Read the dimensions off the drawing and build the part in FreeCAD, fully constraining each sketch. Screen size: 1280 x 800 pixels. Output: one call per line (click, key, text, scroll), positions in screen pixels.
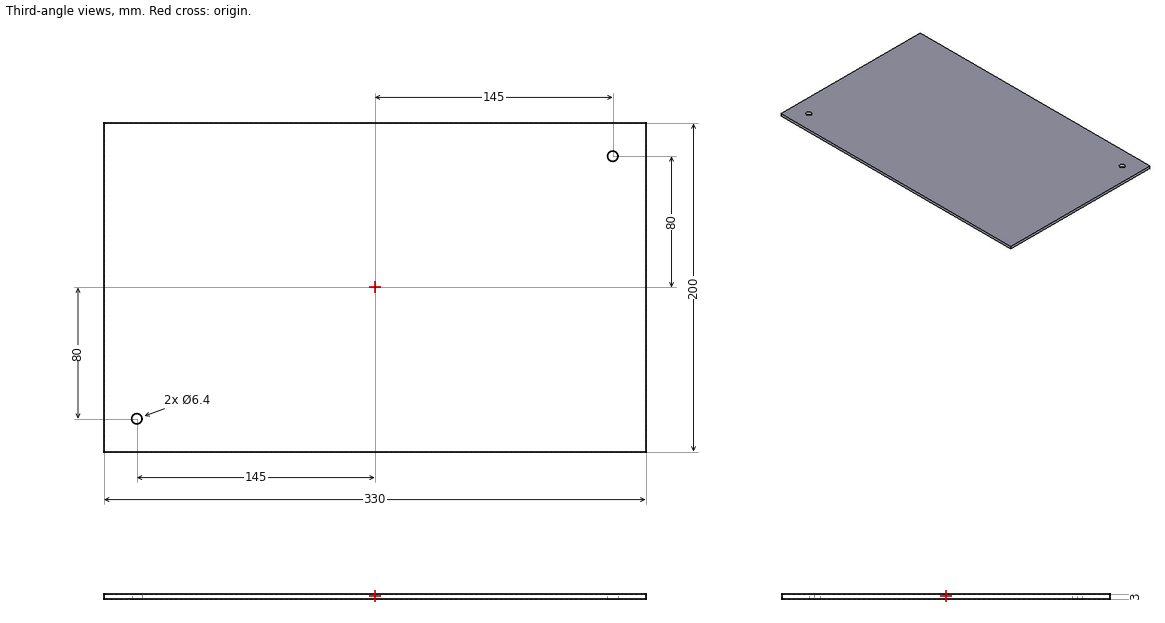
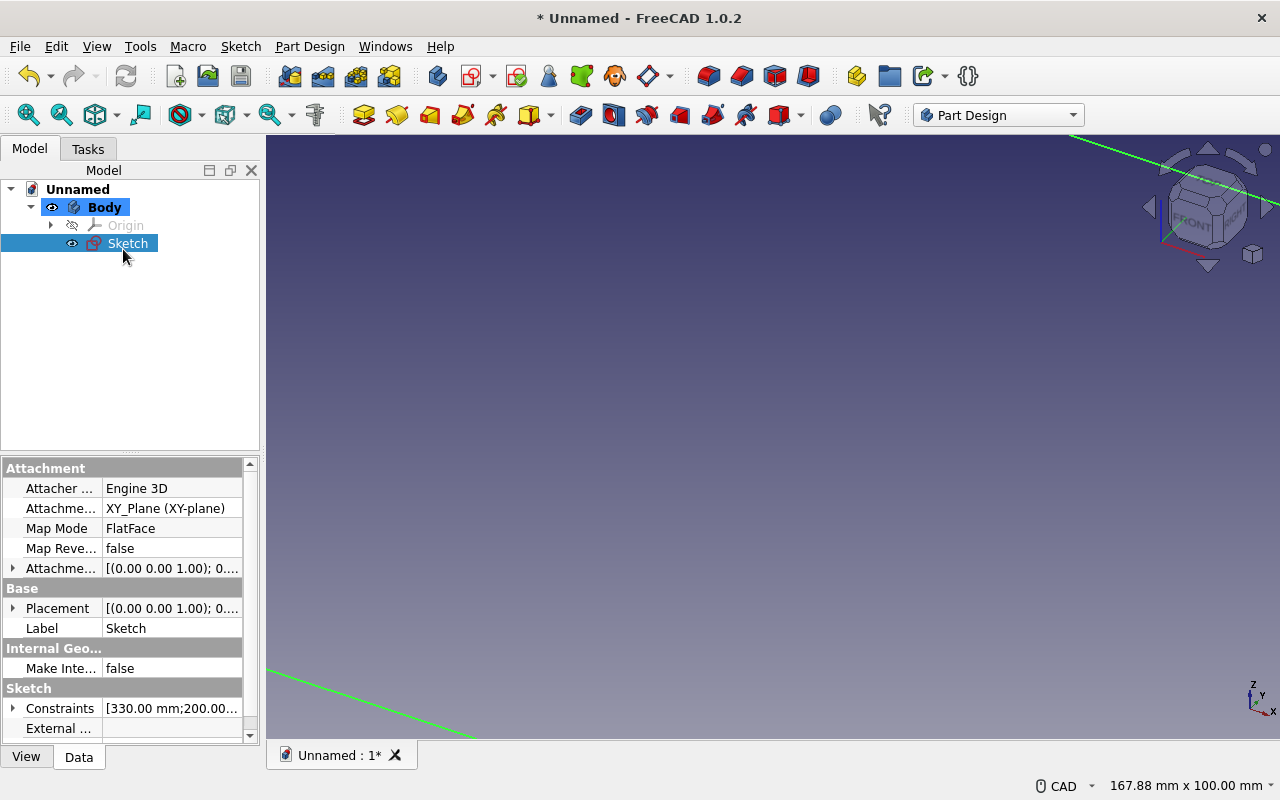
click(364, 116)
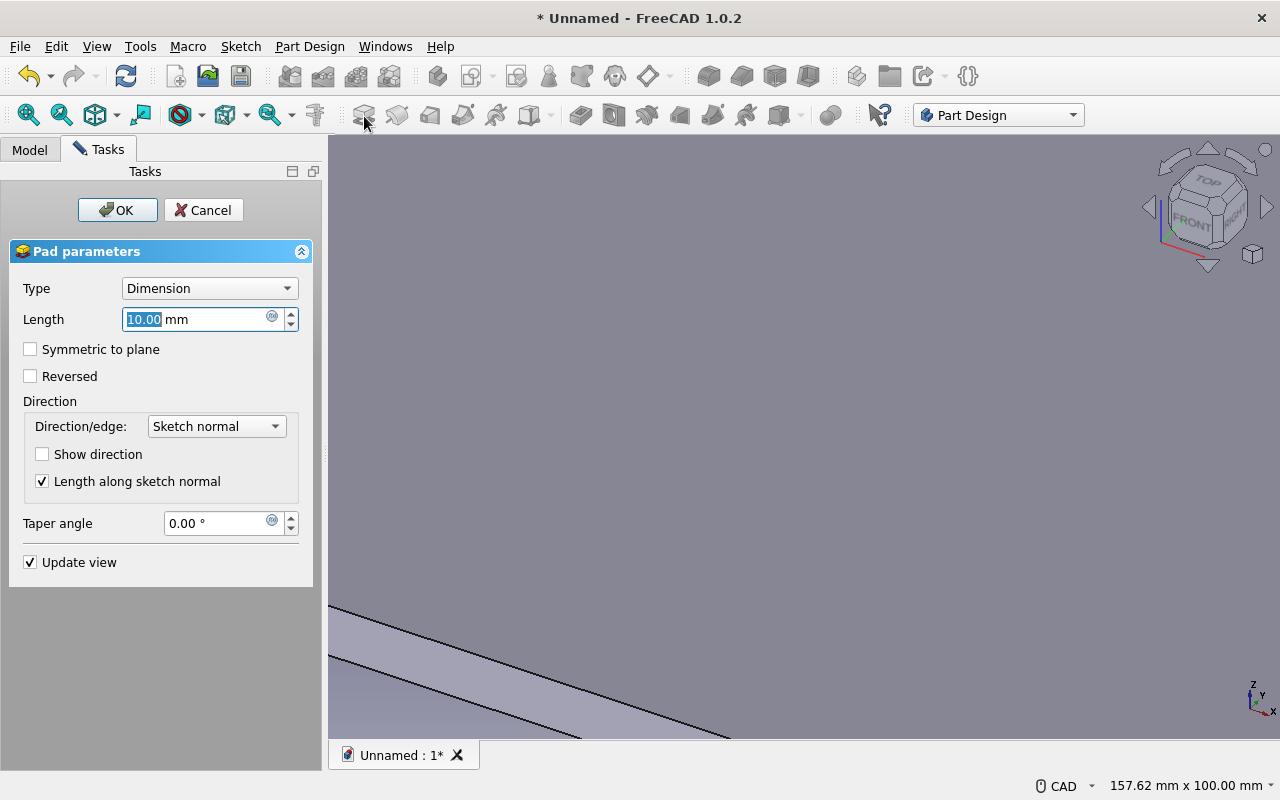
text(3)
key(Tab)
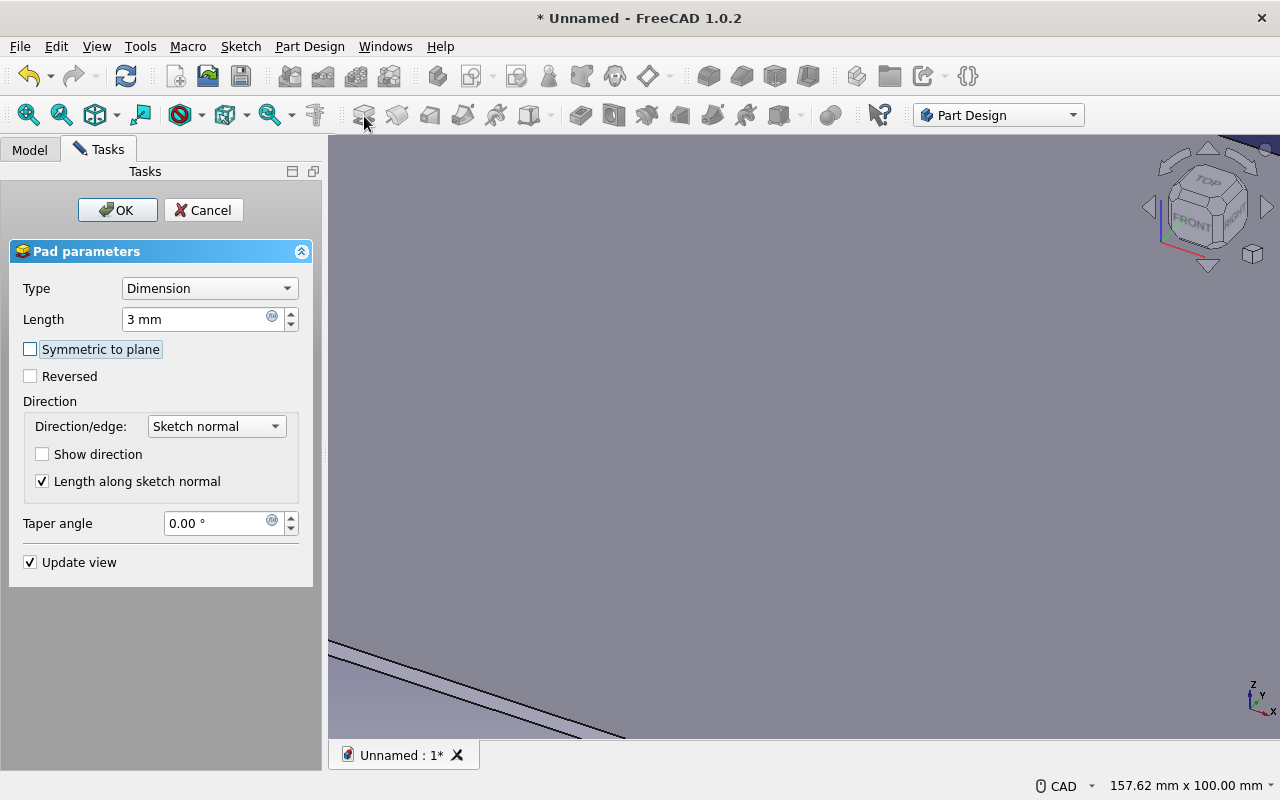
click(31, 349)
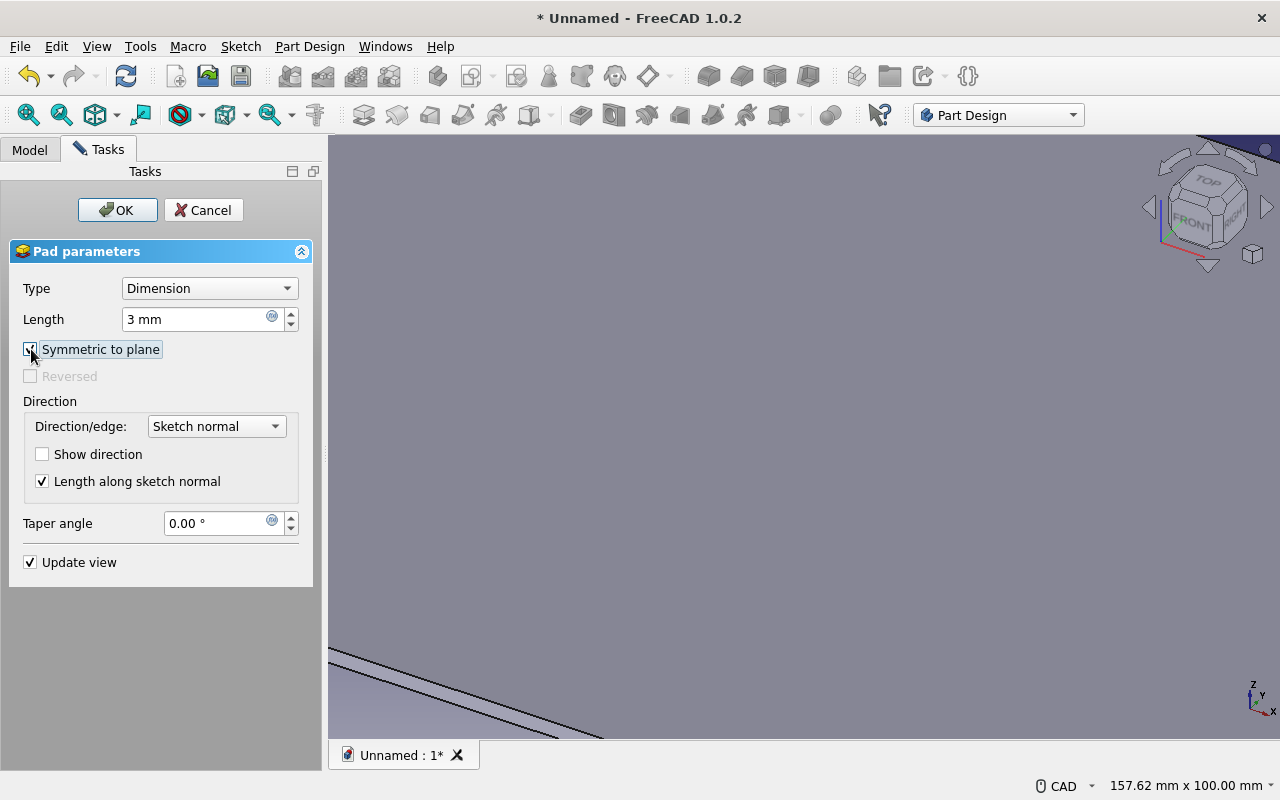
click(118, 210)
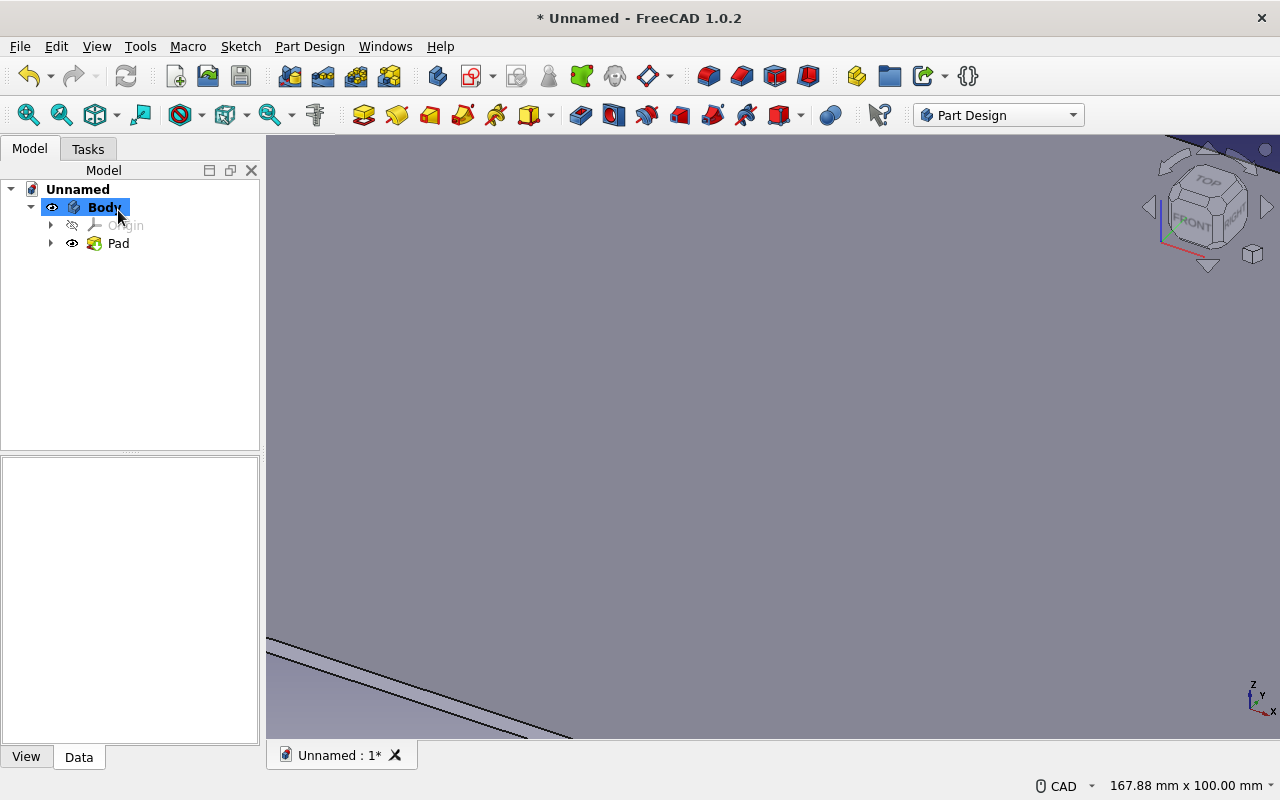
click(29, 116)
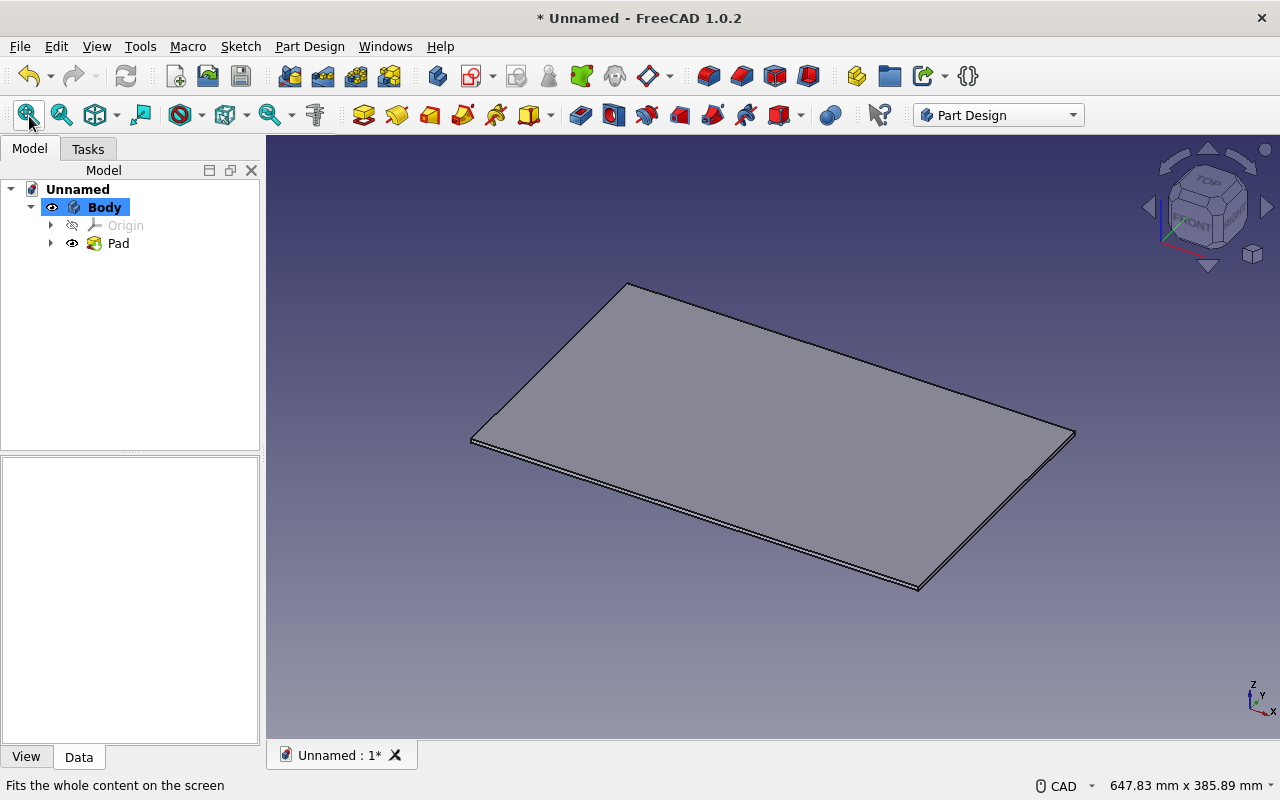
click(470, 76)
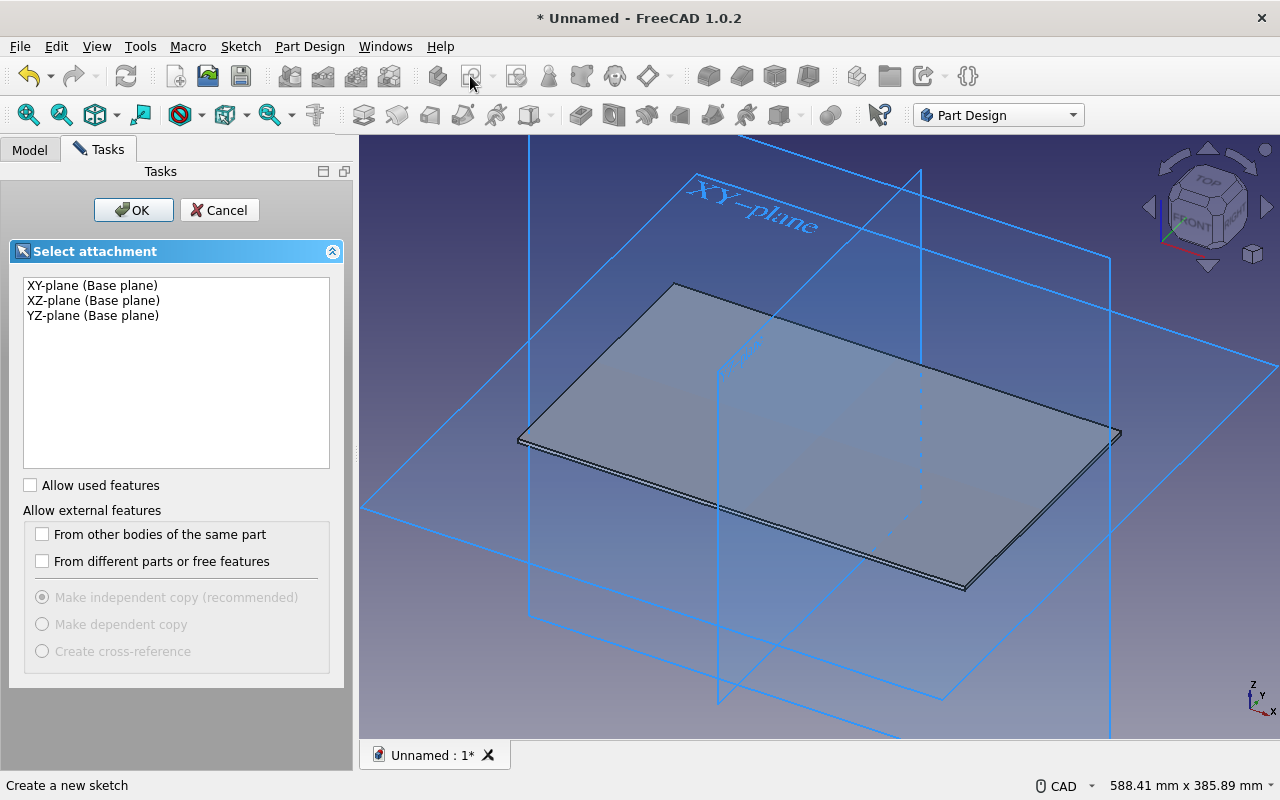
click(84, 286)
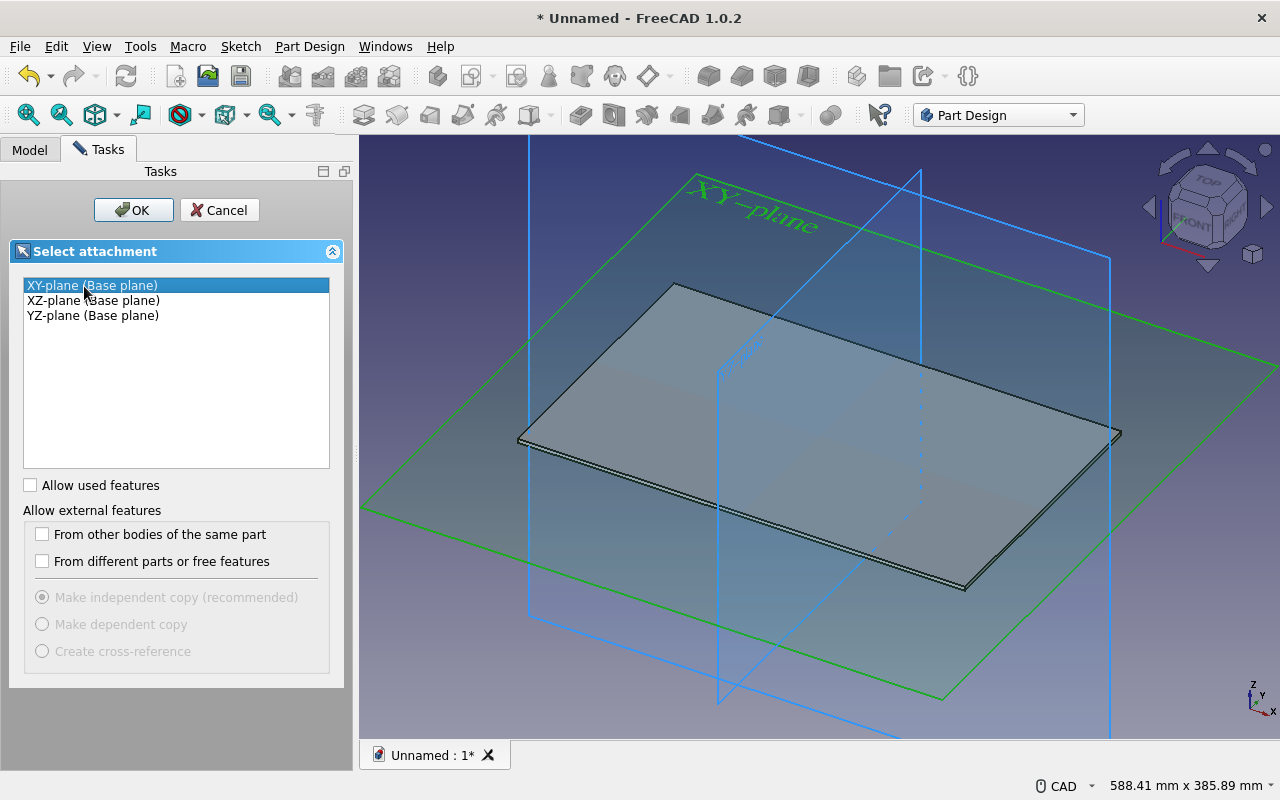
click(134, 210)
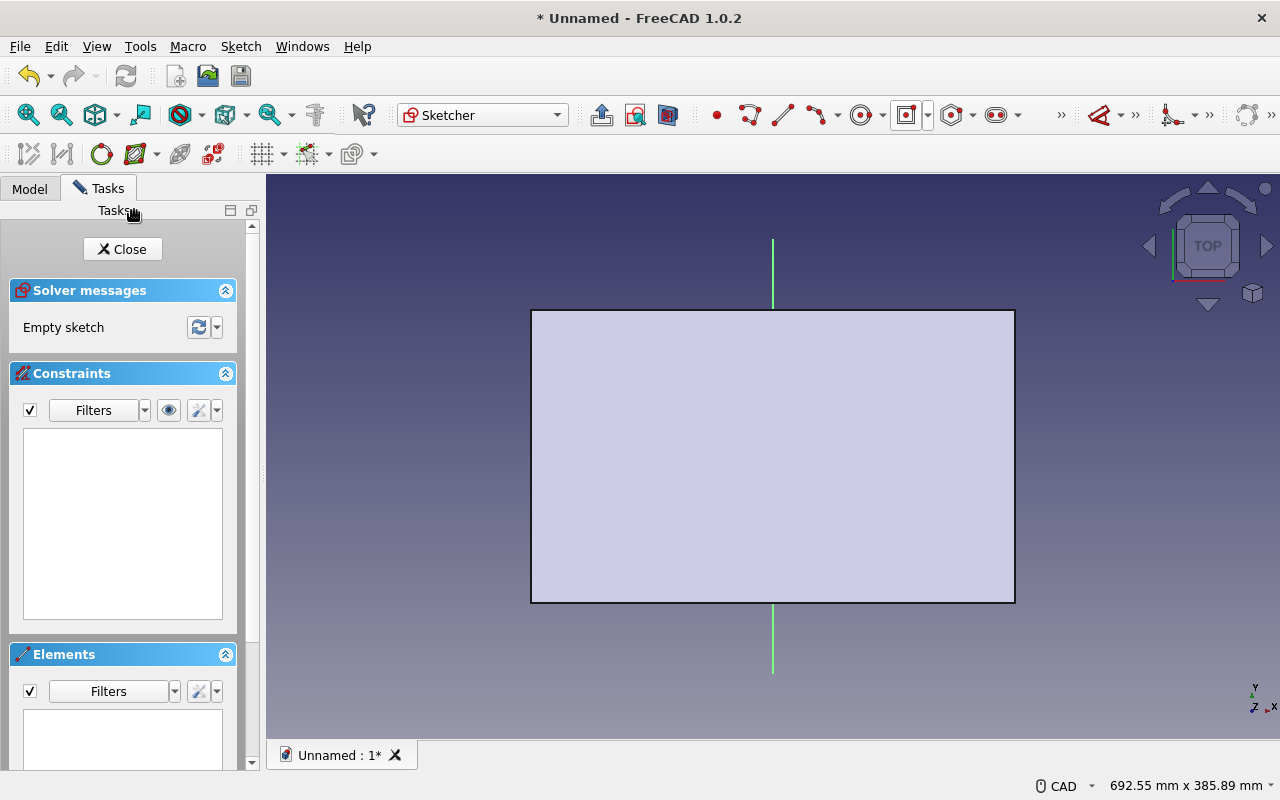
click(668, 116)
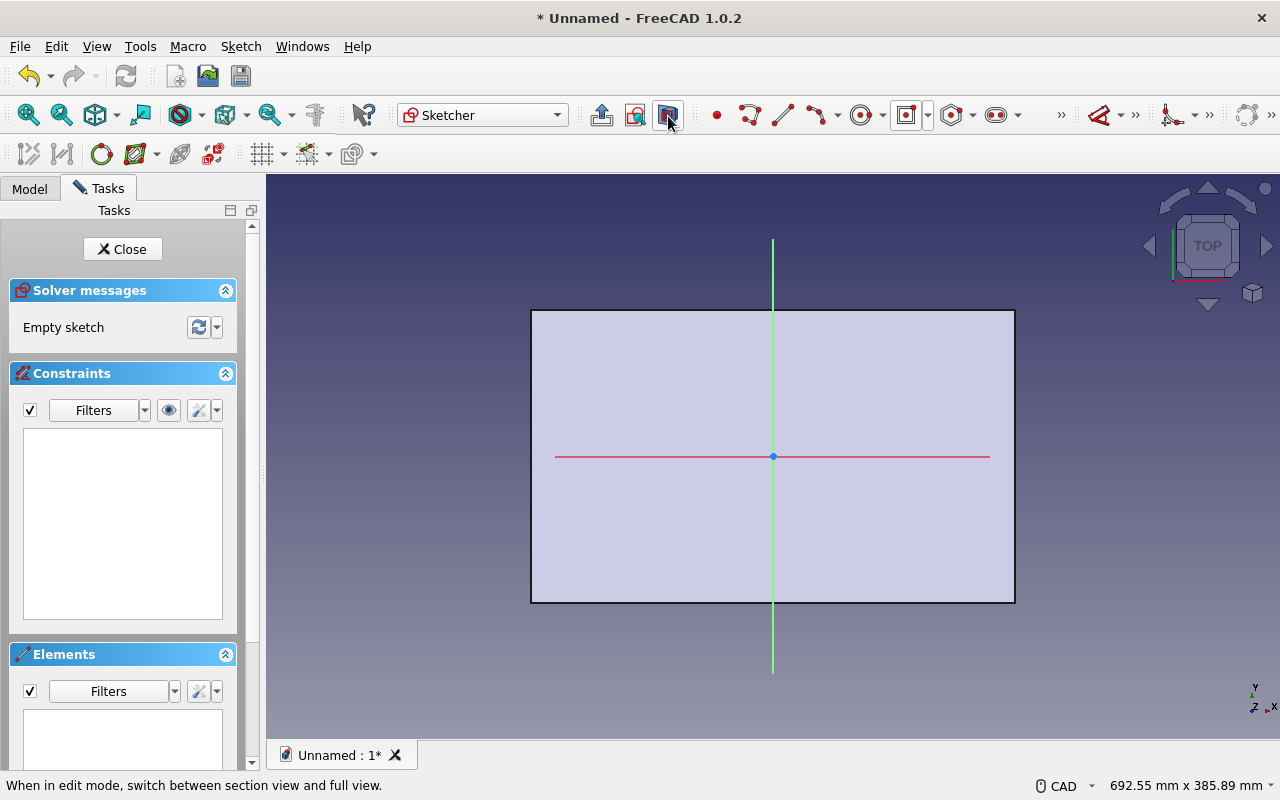
click(860, 116)